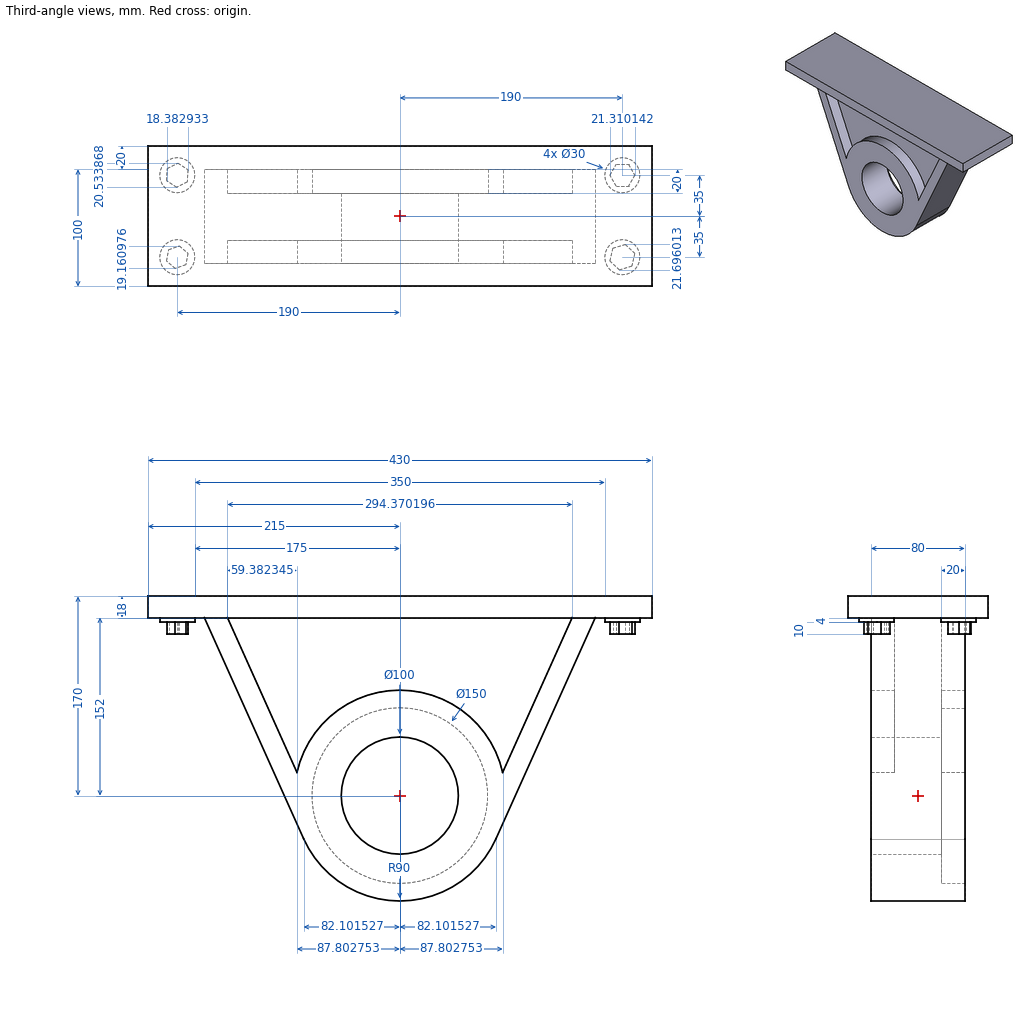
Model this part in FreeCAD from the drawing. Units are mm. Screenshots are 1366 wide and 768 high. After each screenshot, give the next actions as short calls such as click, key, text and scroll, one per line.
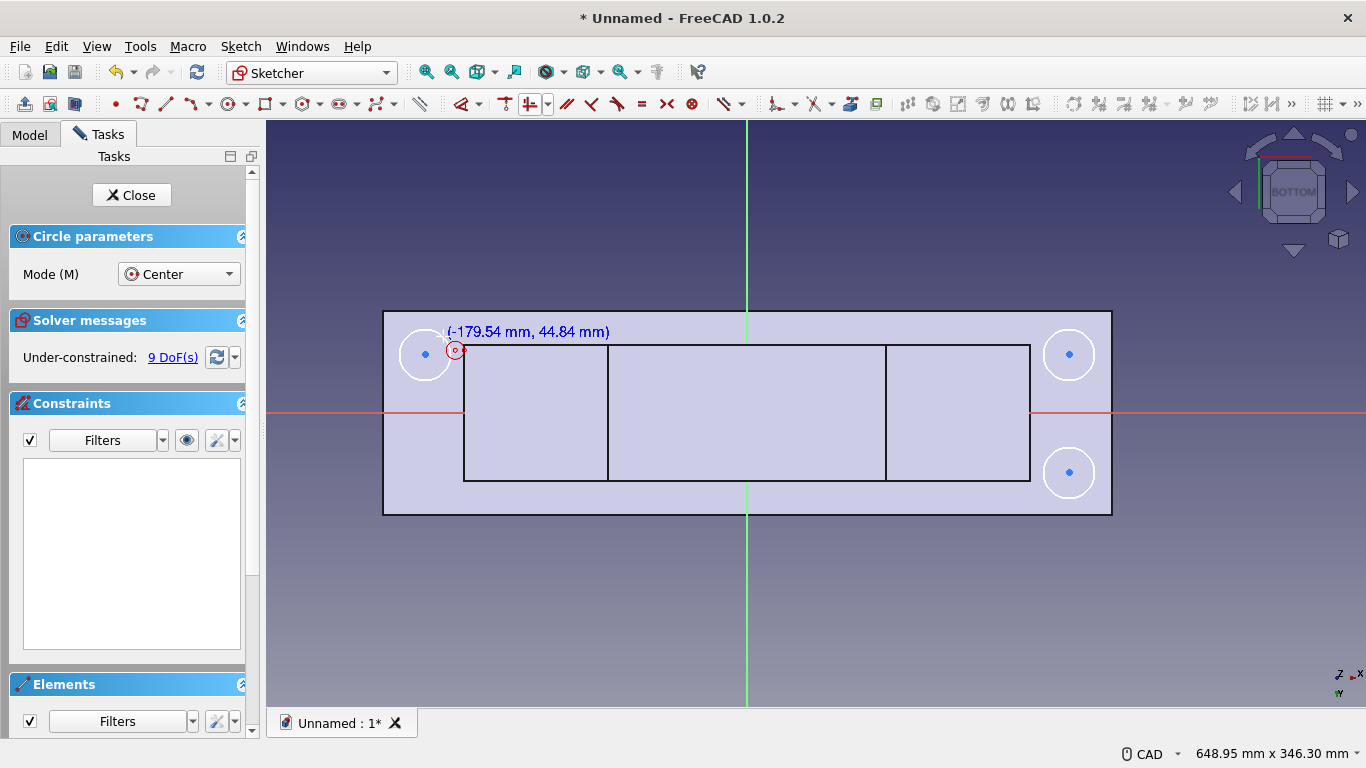
click(425, 472)
click(443, 454)
key(Escape)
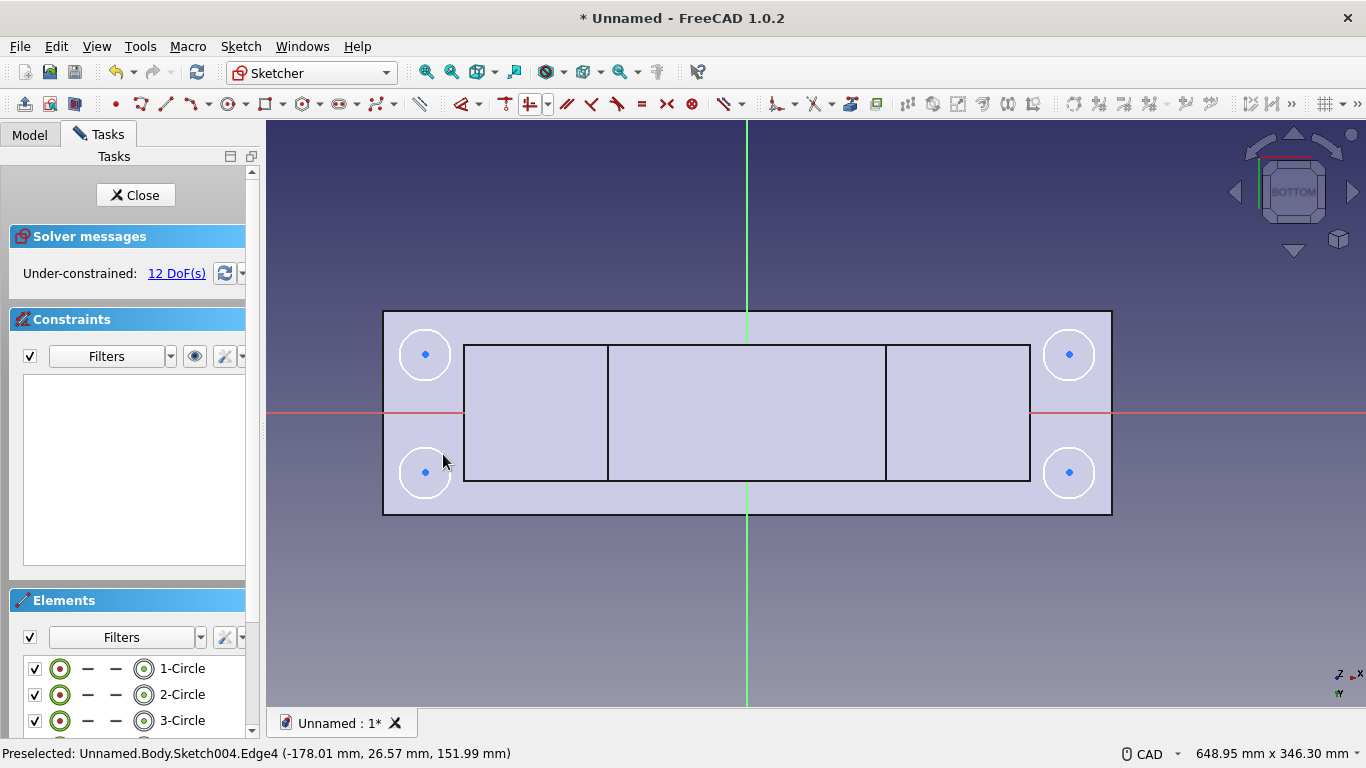
click(1087, 455)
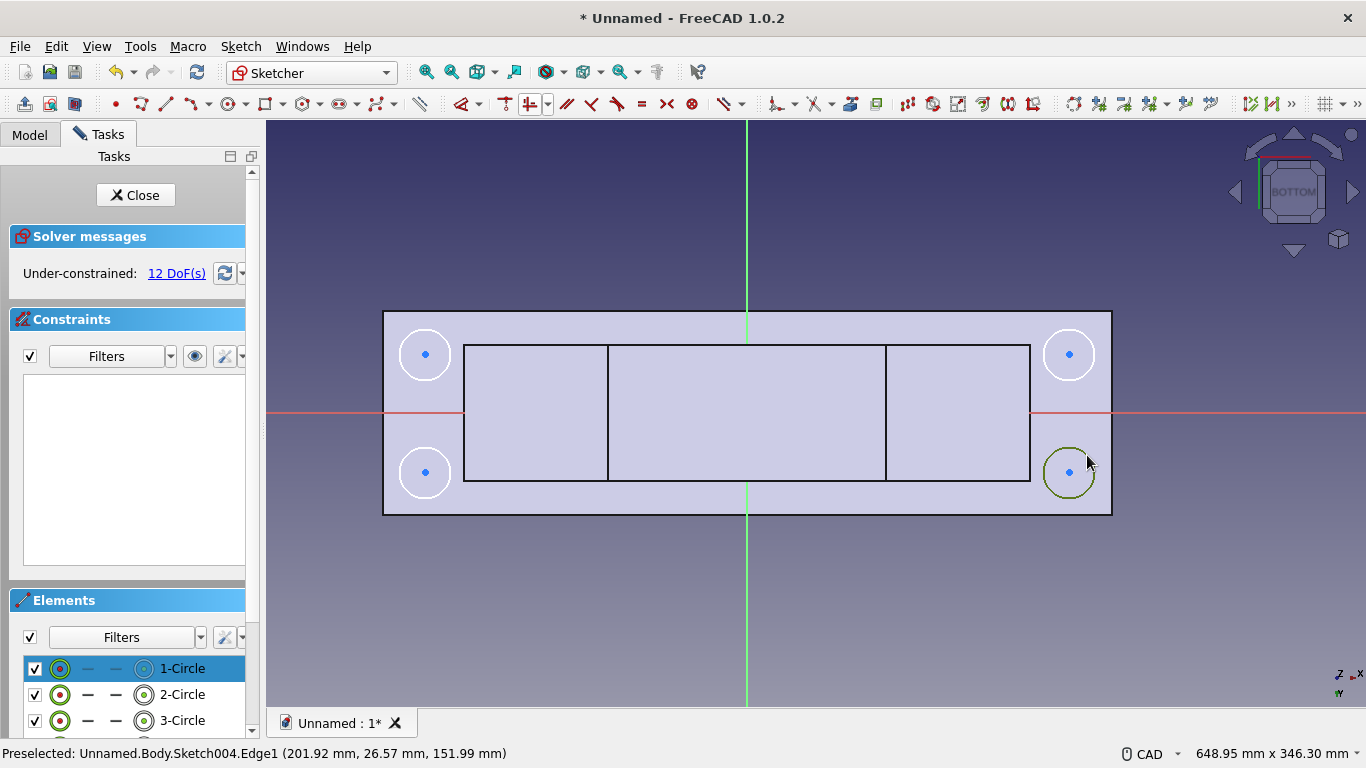
click(1087, 337)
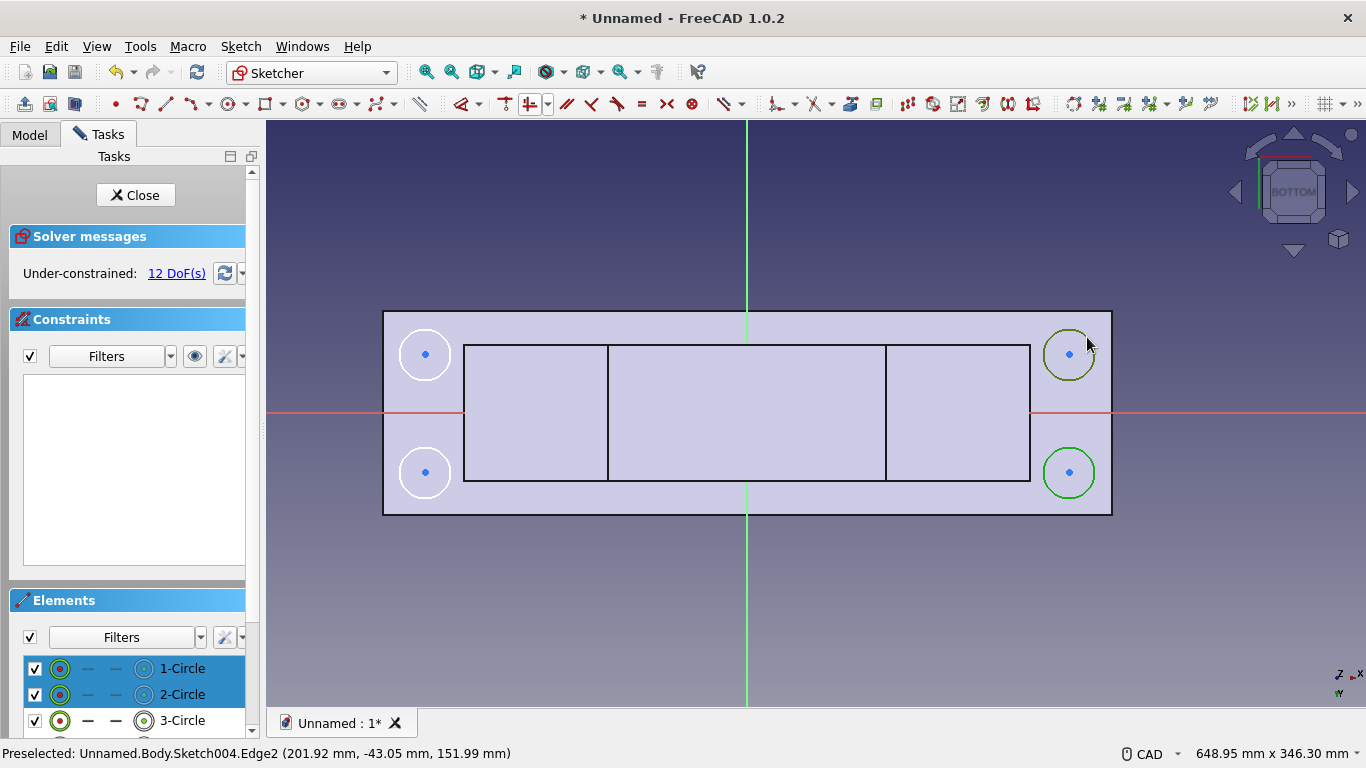
click(443, 337)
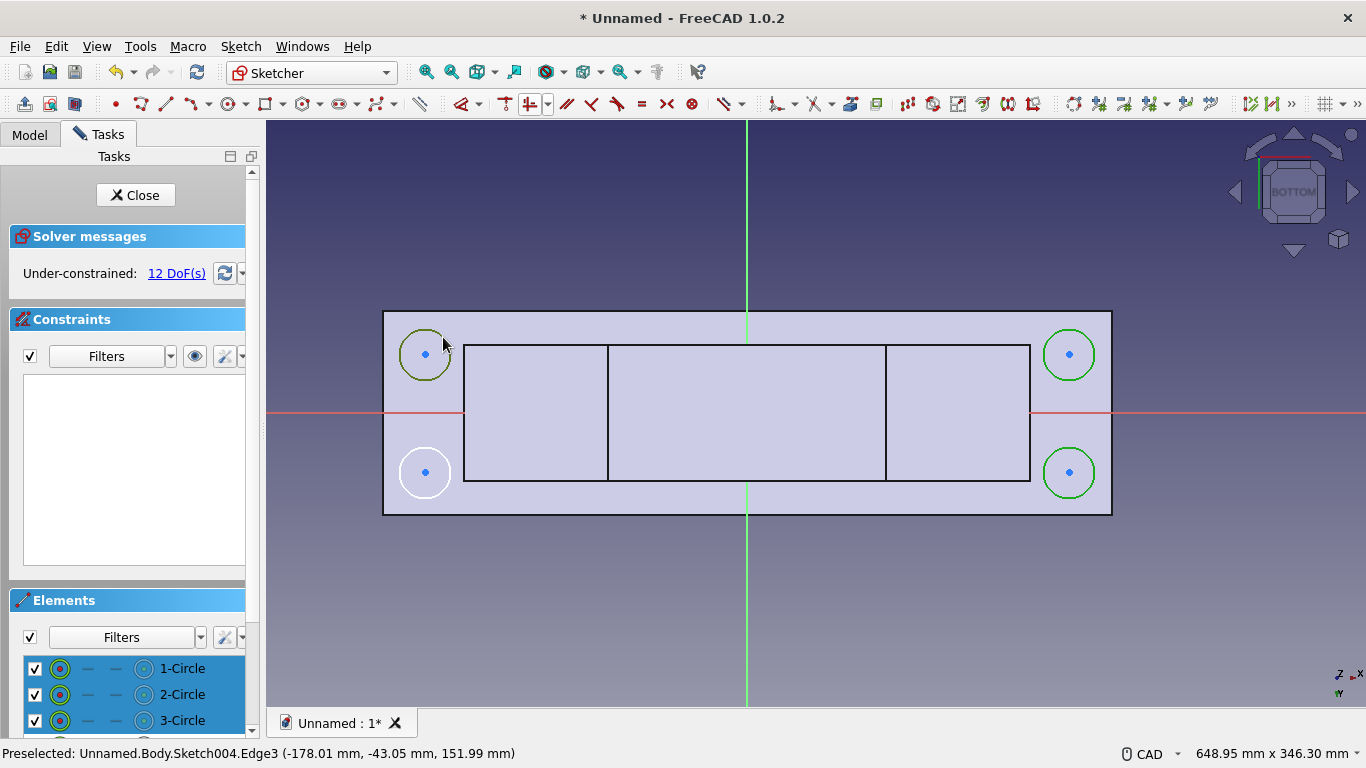
click(443, 455)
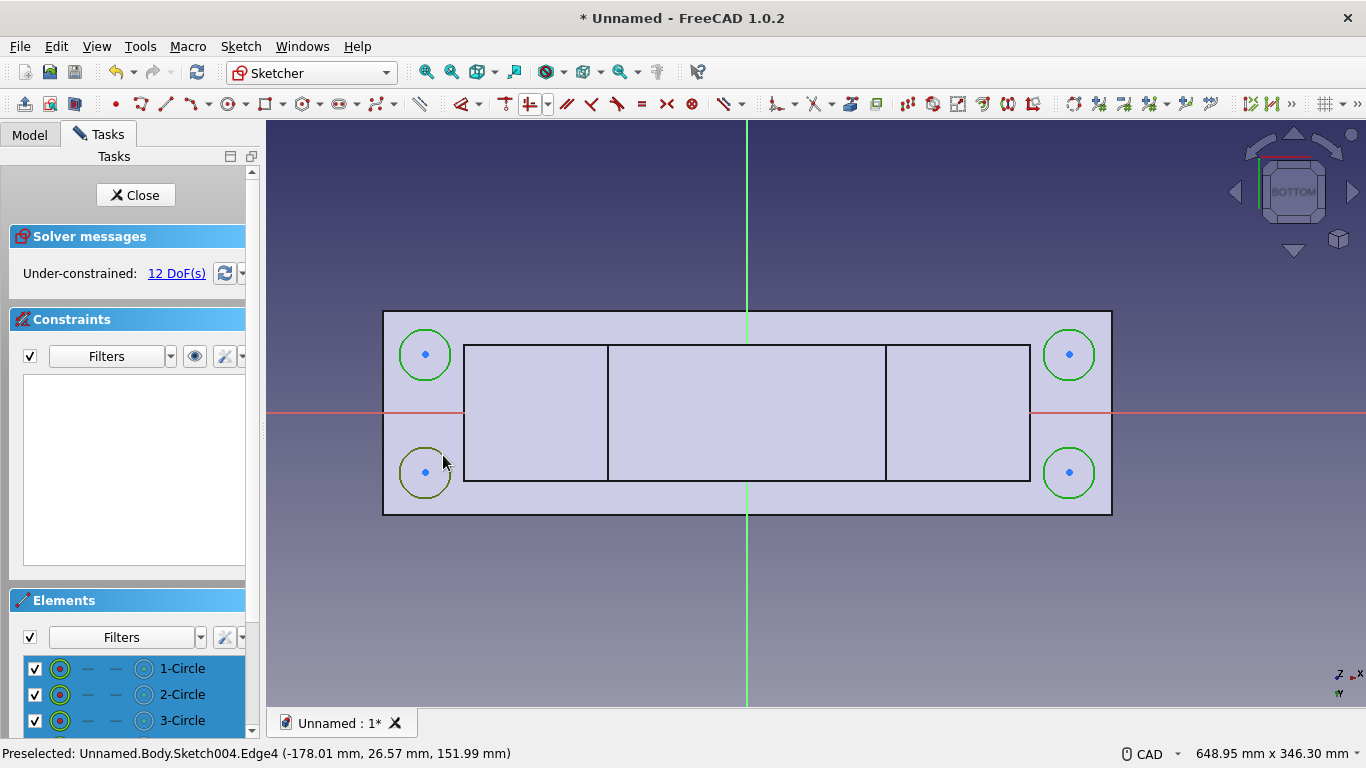
click(642, 104)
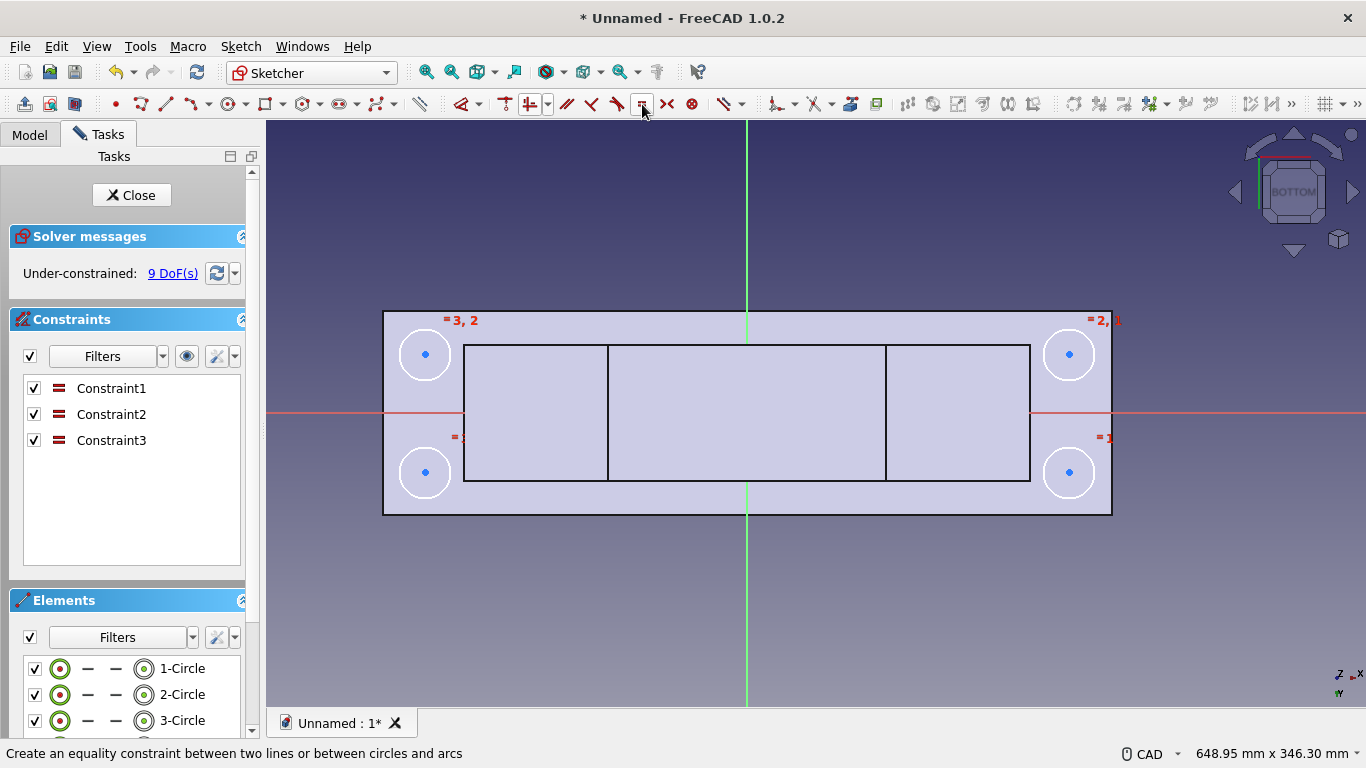
click(460, 104)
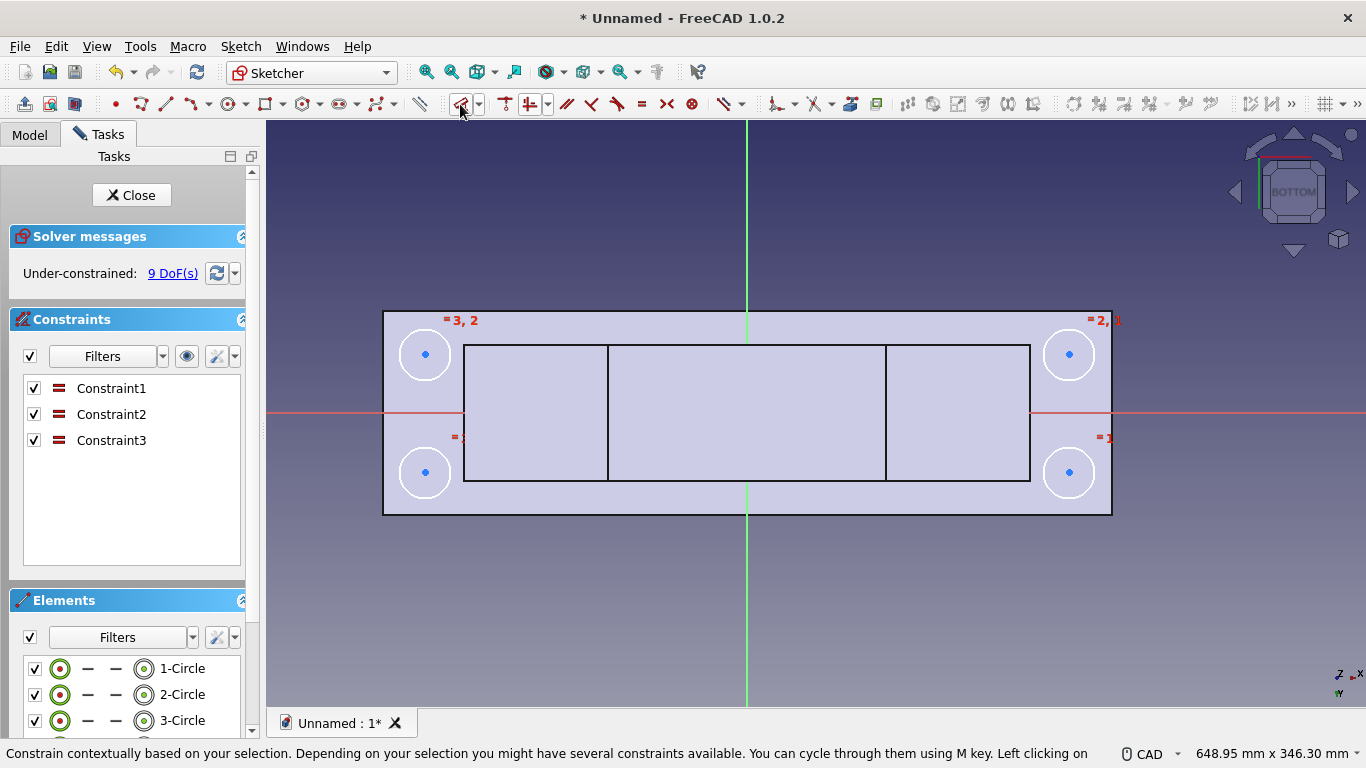
click(1087, 455)
click(1110, 432)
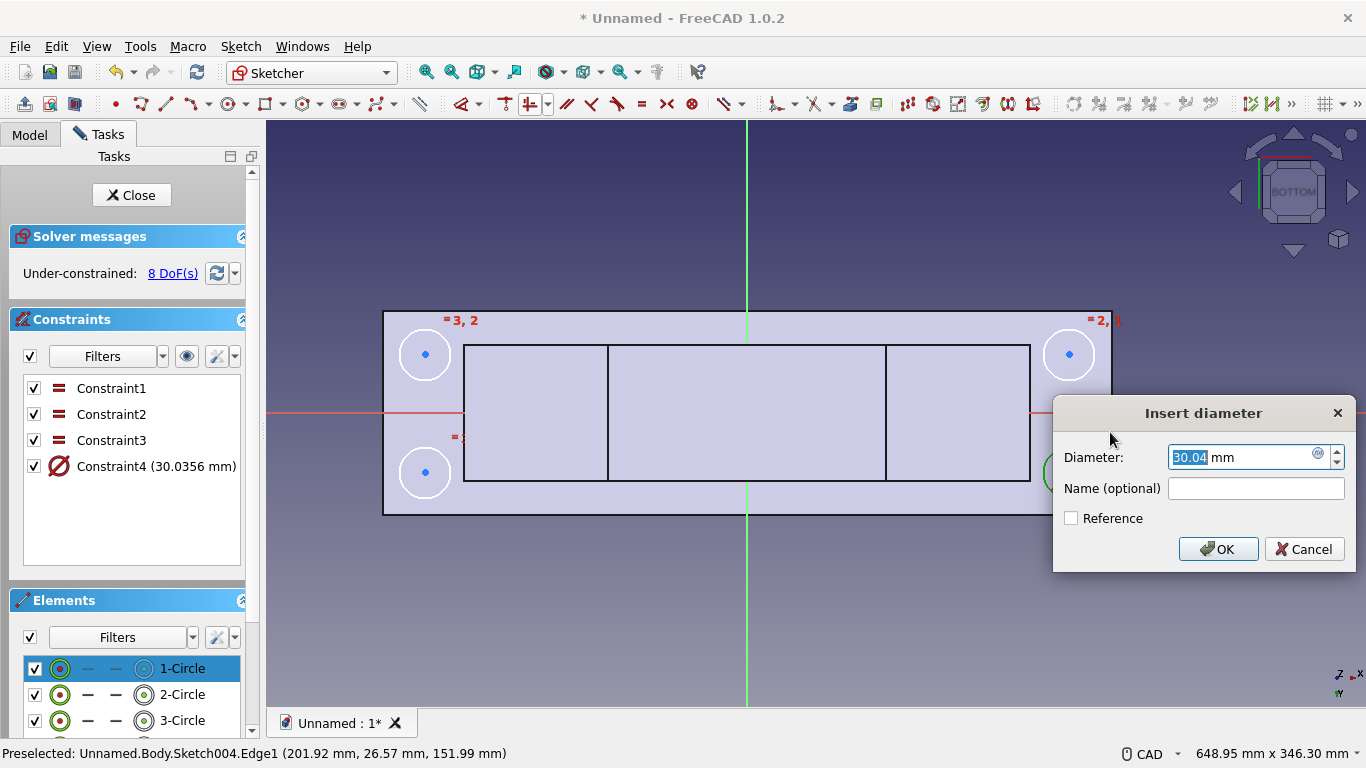
text(30)
key(Return)